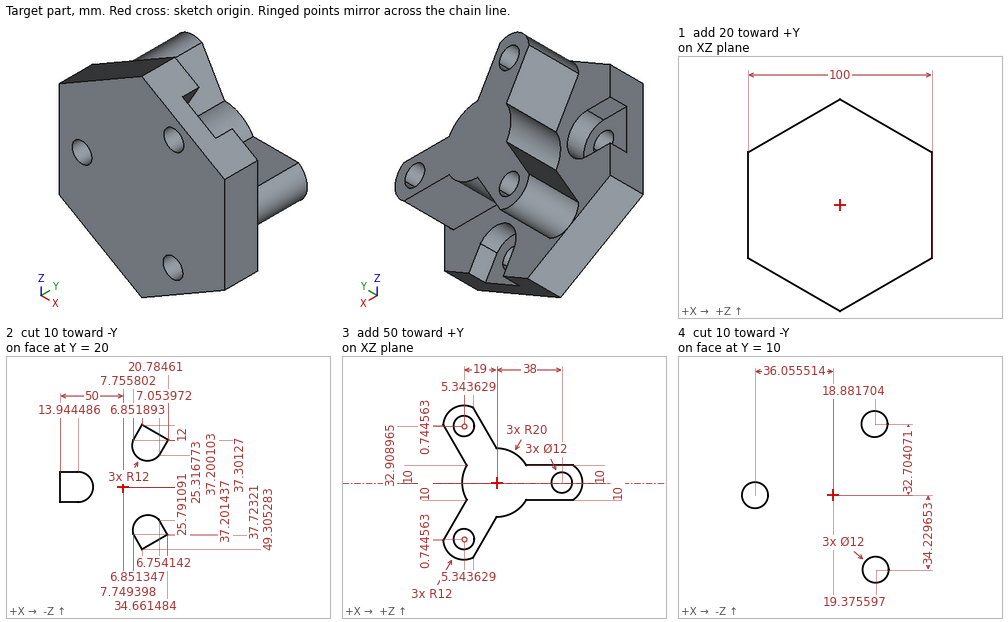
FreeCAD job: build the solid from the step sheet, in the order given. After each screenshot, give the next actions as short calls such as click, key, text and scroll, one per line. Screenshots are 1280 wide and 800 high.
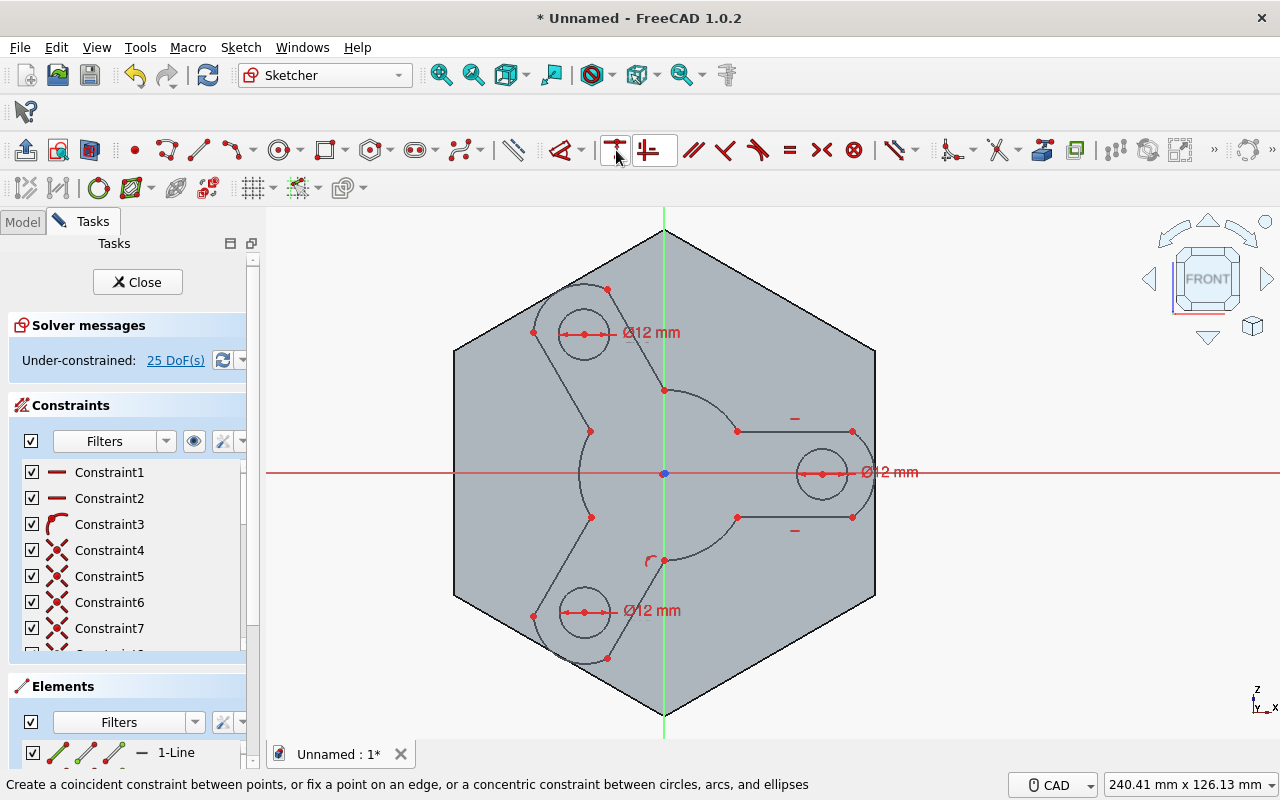
click(691, 556)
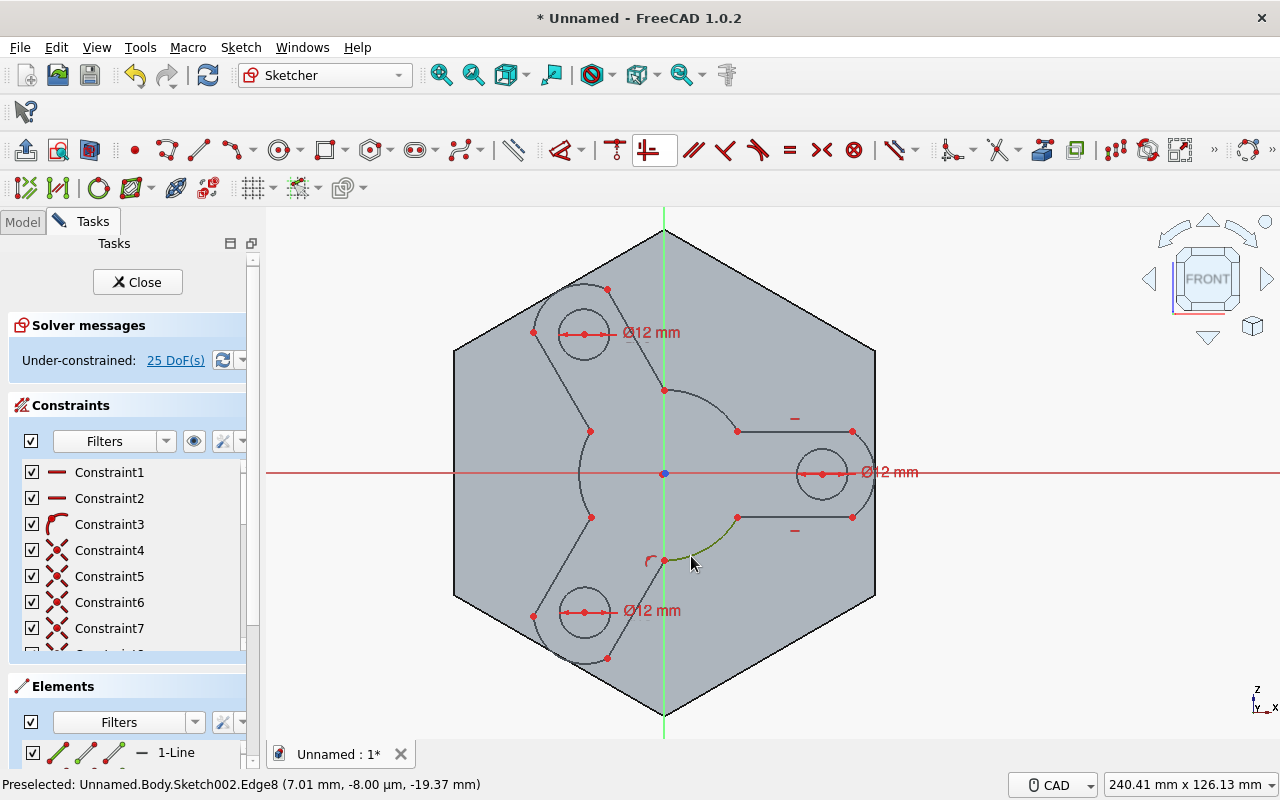
click(721, 411)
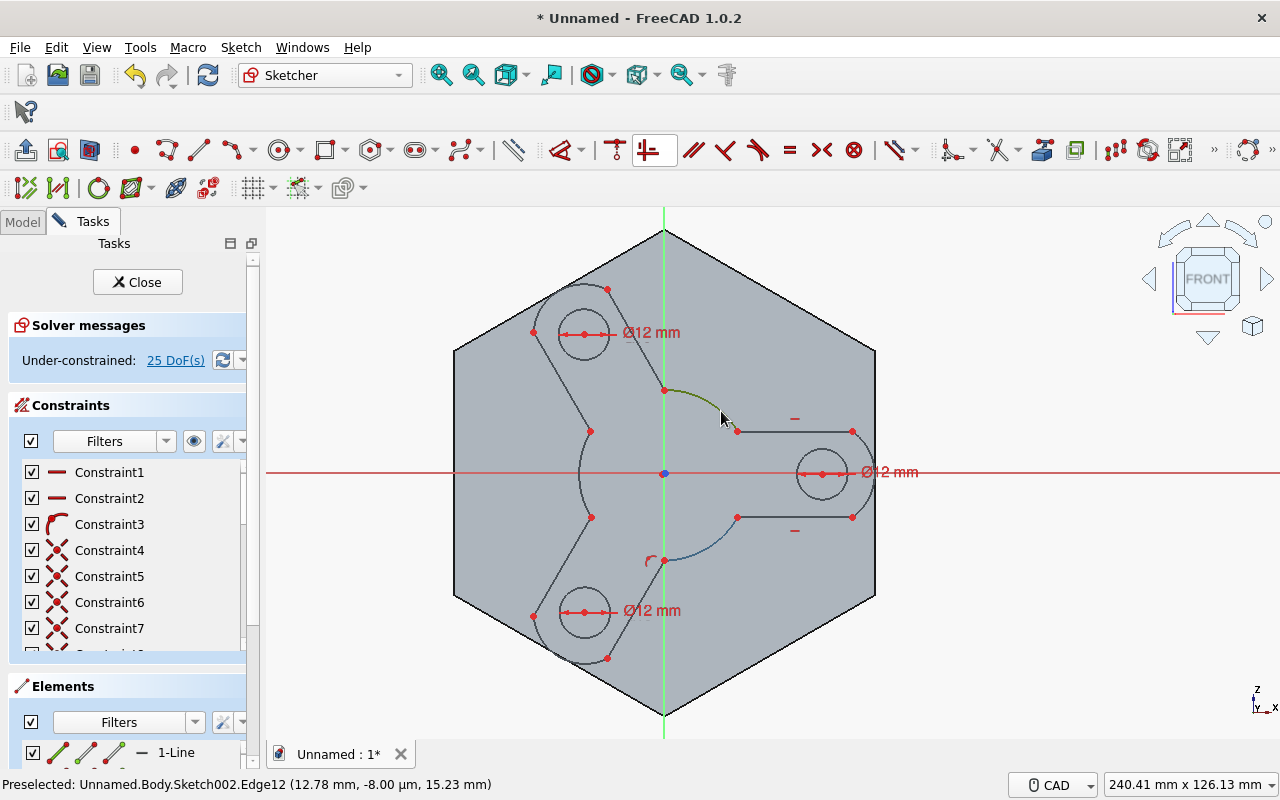
click(616, 150)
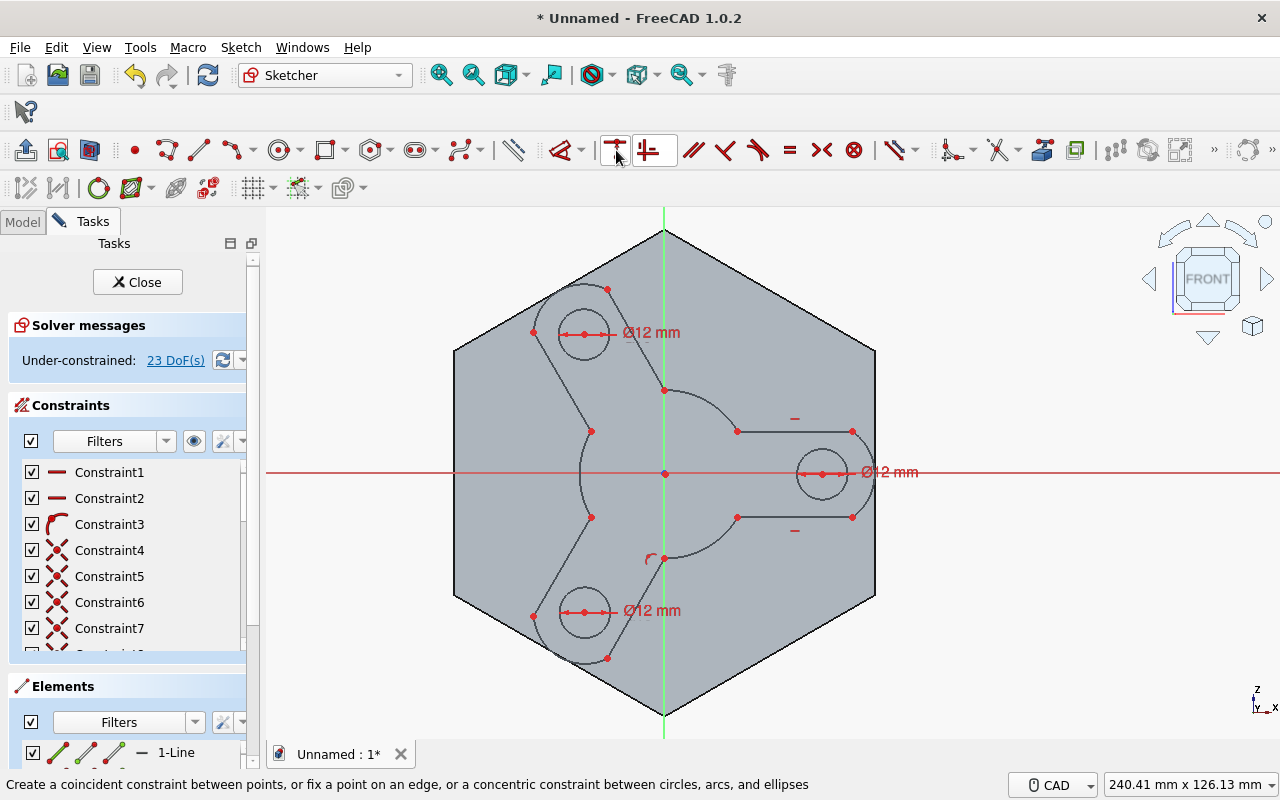
scroll(665, 474, up, 3)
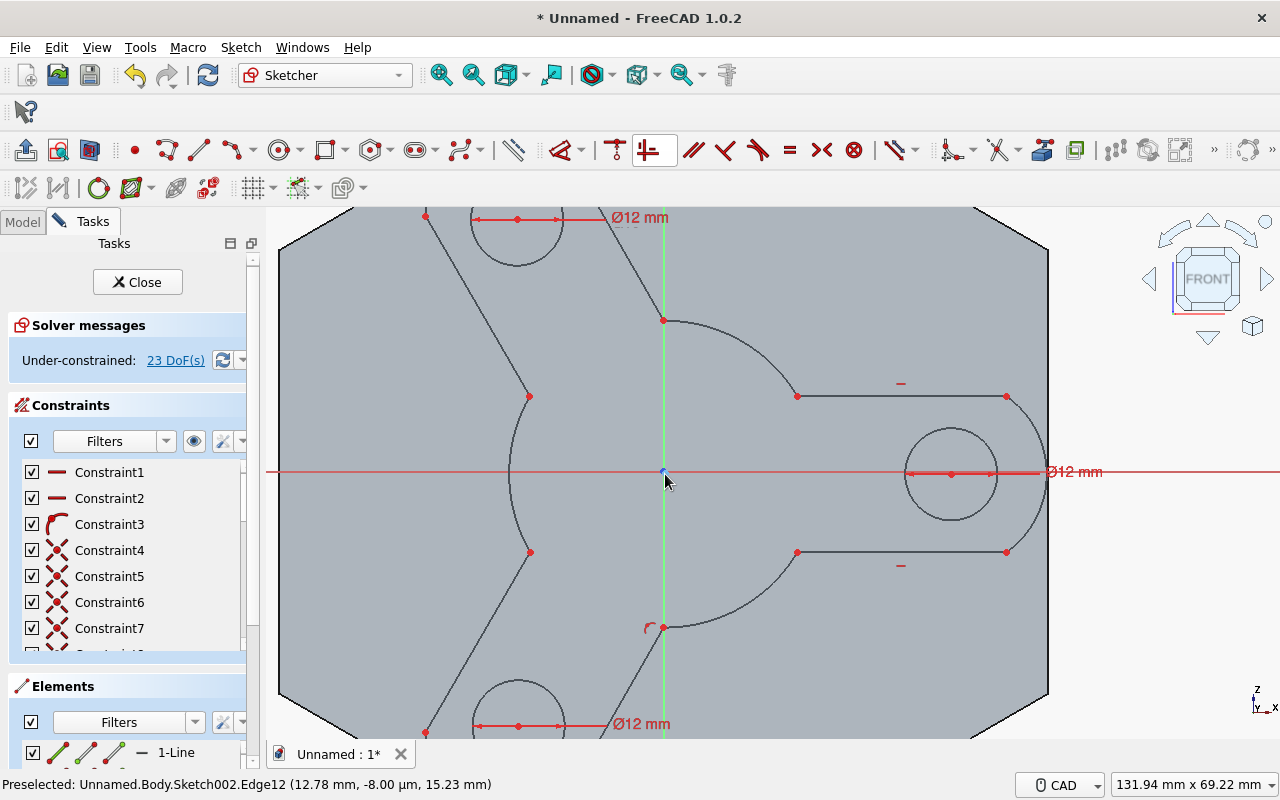
drag(654, 462, 675, 484)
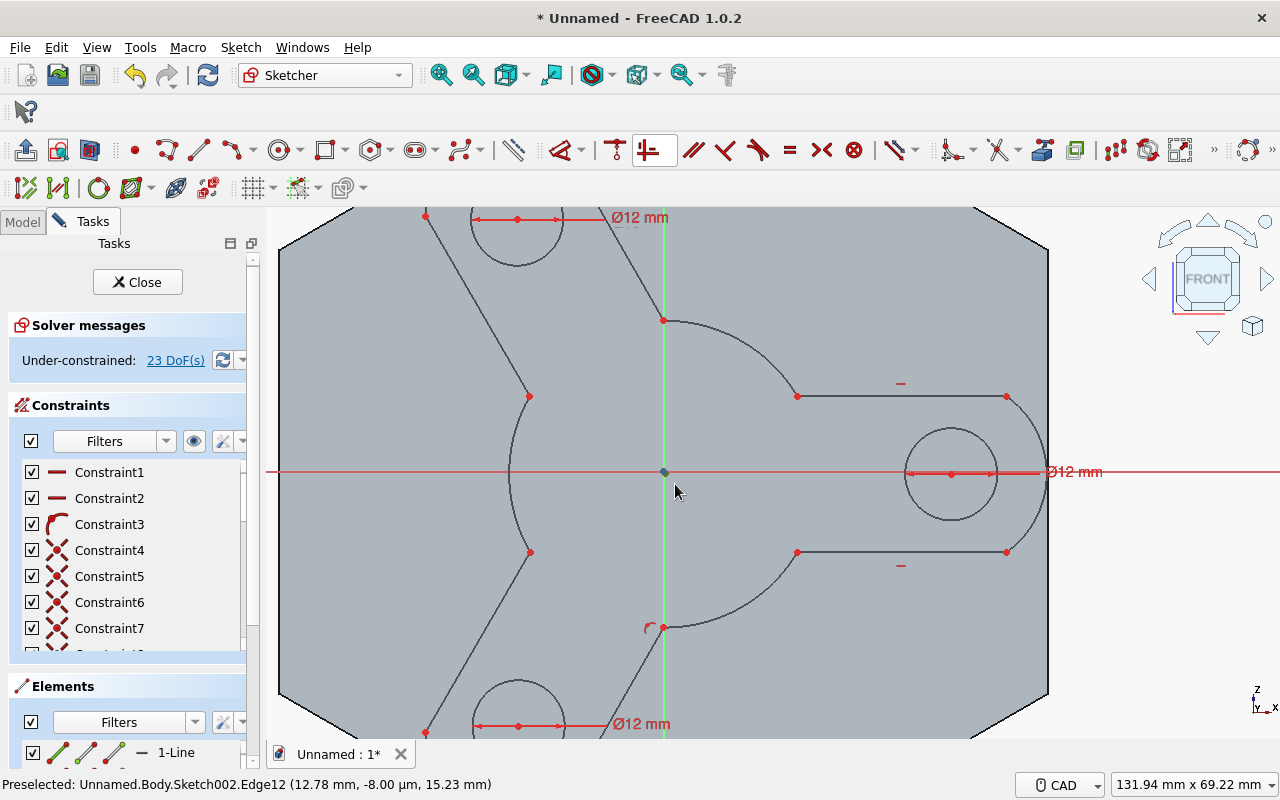
click(616, 150)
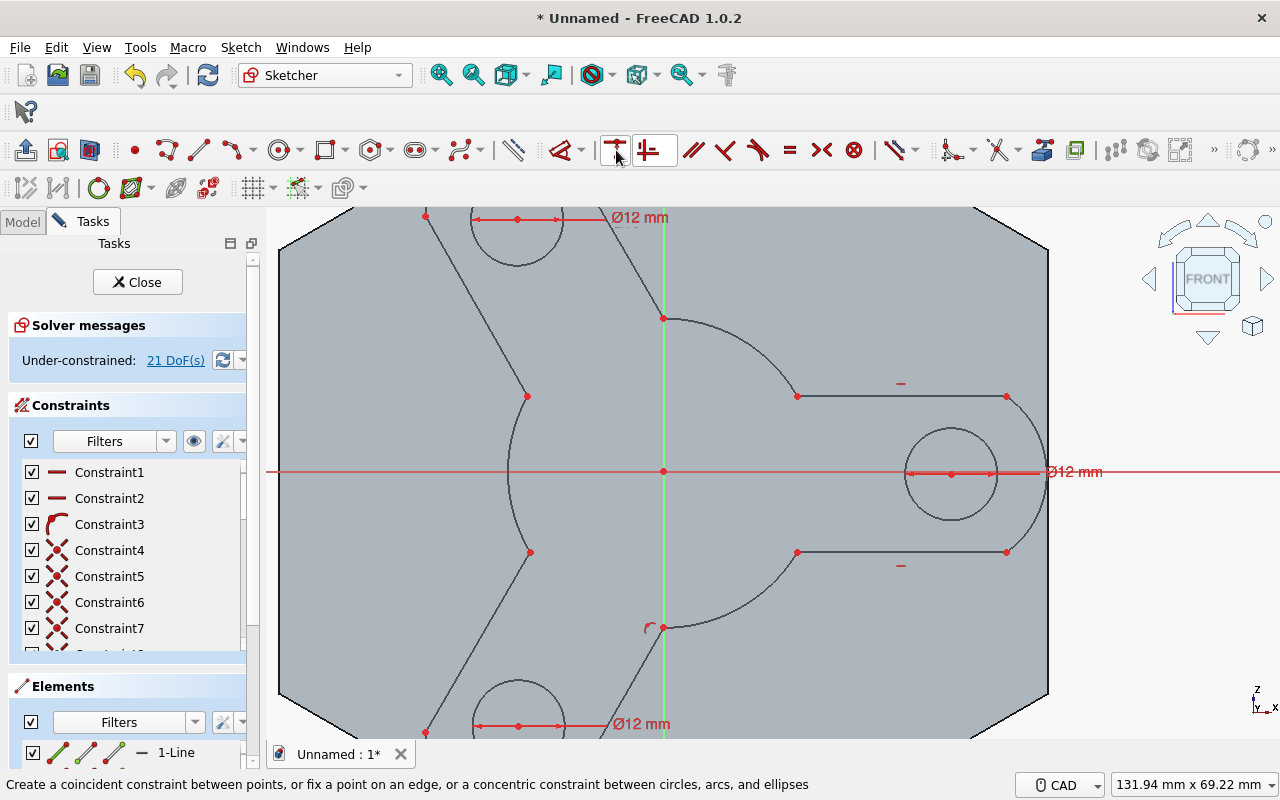
click(1040, 510)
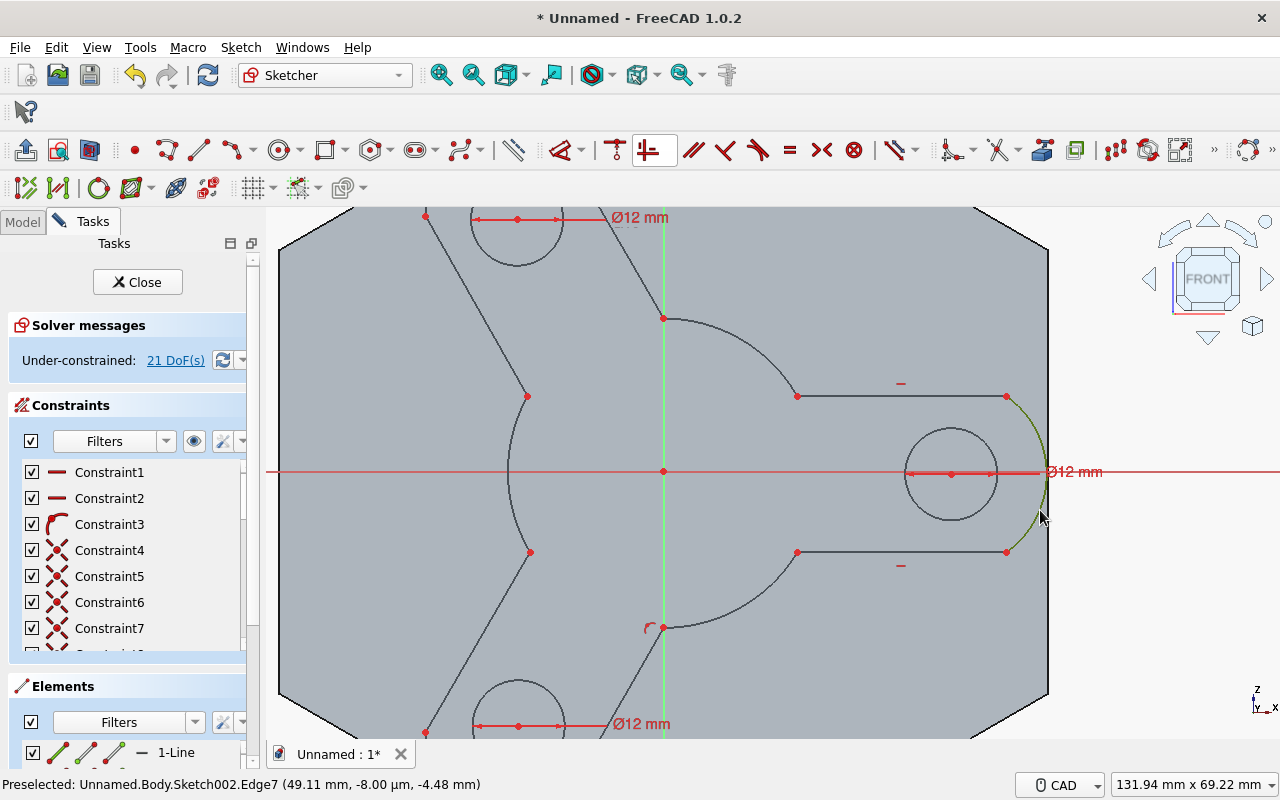
scroll(665, 474, down, 3)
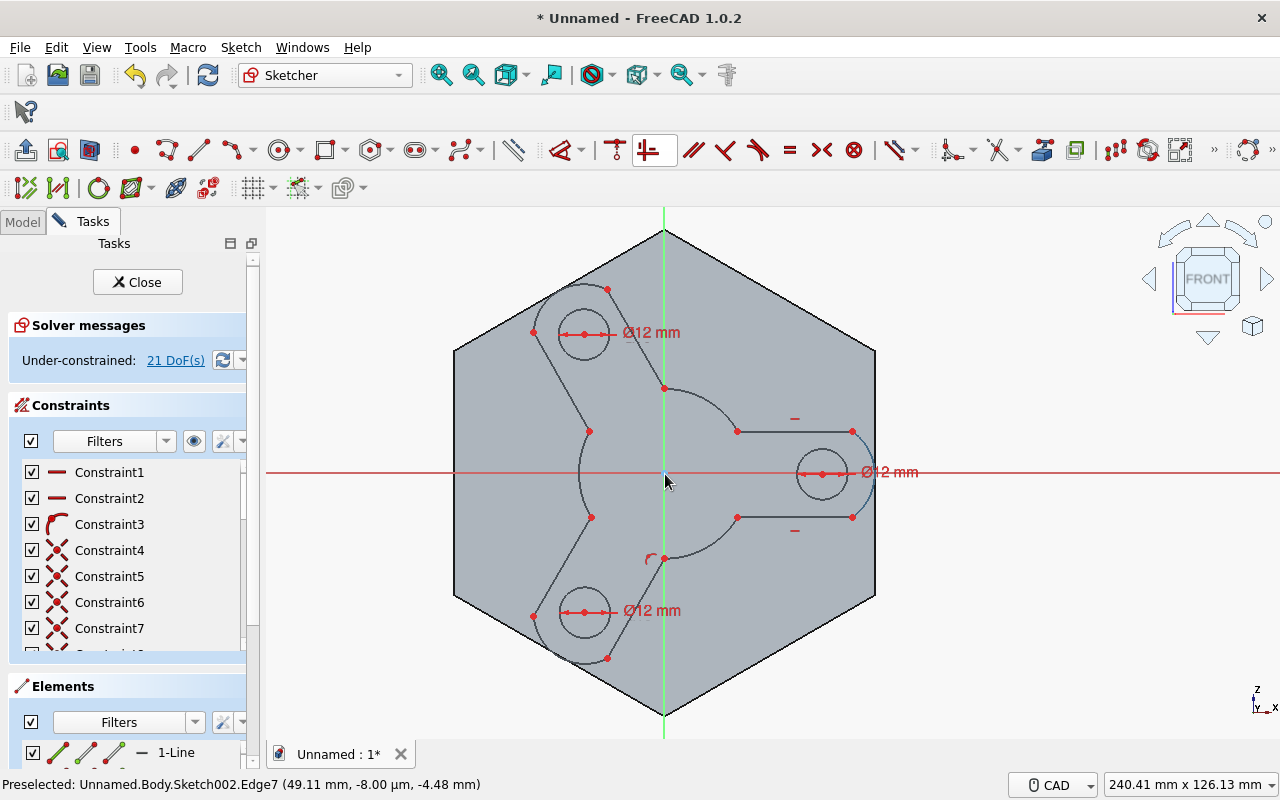
click(544, 644)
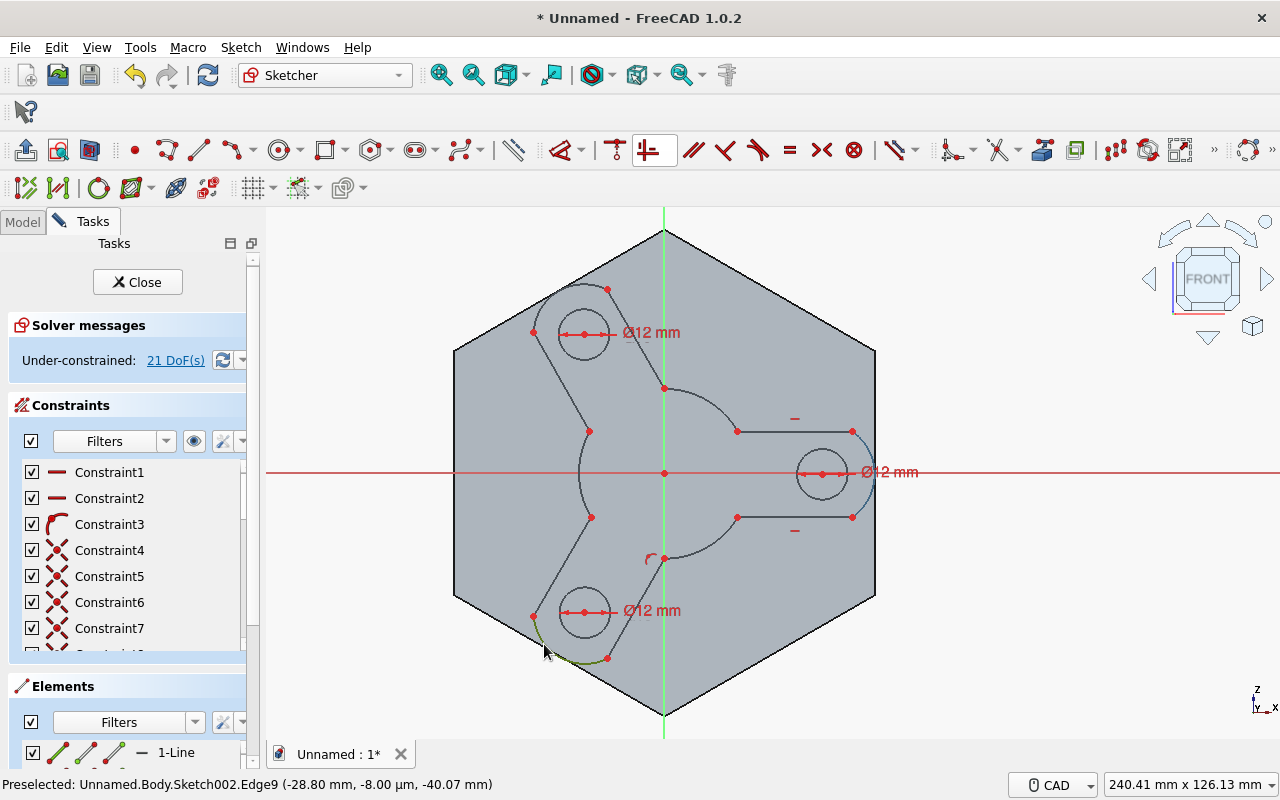
click(578, 285)